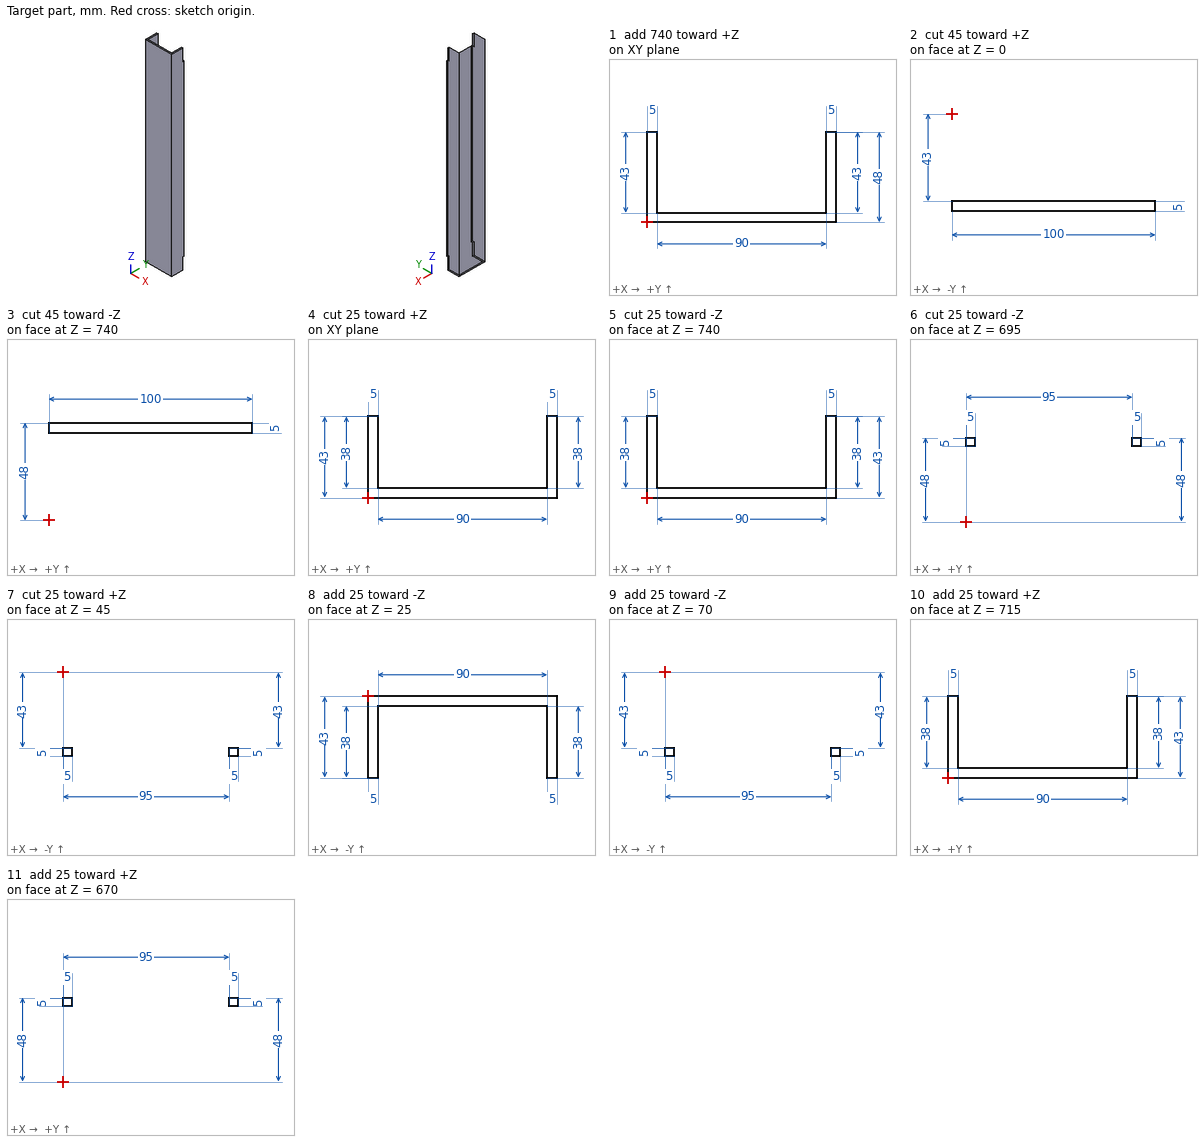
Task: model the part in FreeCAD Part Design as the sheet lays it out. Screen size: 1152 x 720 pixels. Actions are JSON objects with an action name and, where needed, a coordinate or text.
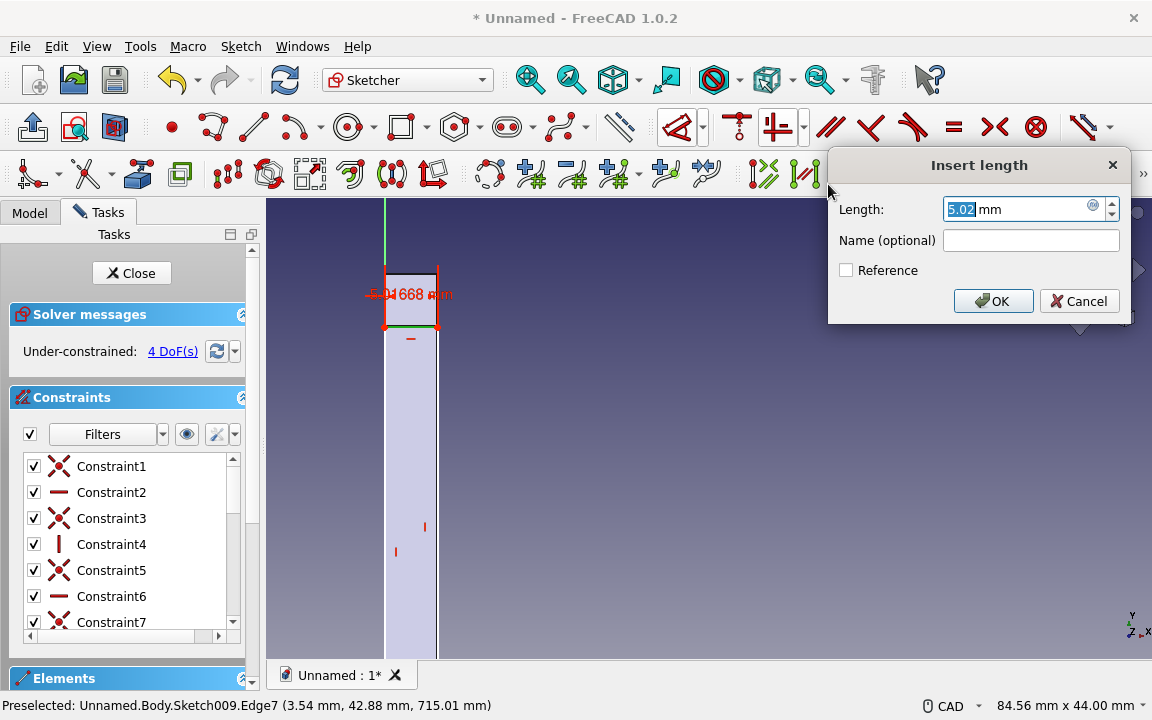
{"action": "type", "text": "5"}
{"action": "key", "text": "Return"}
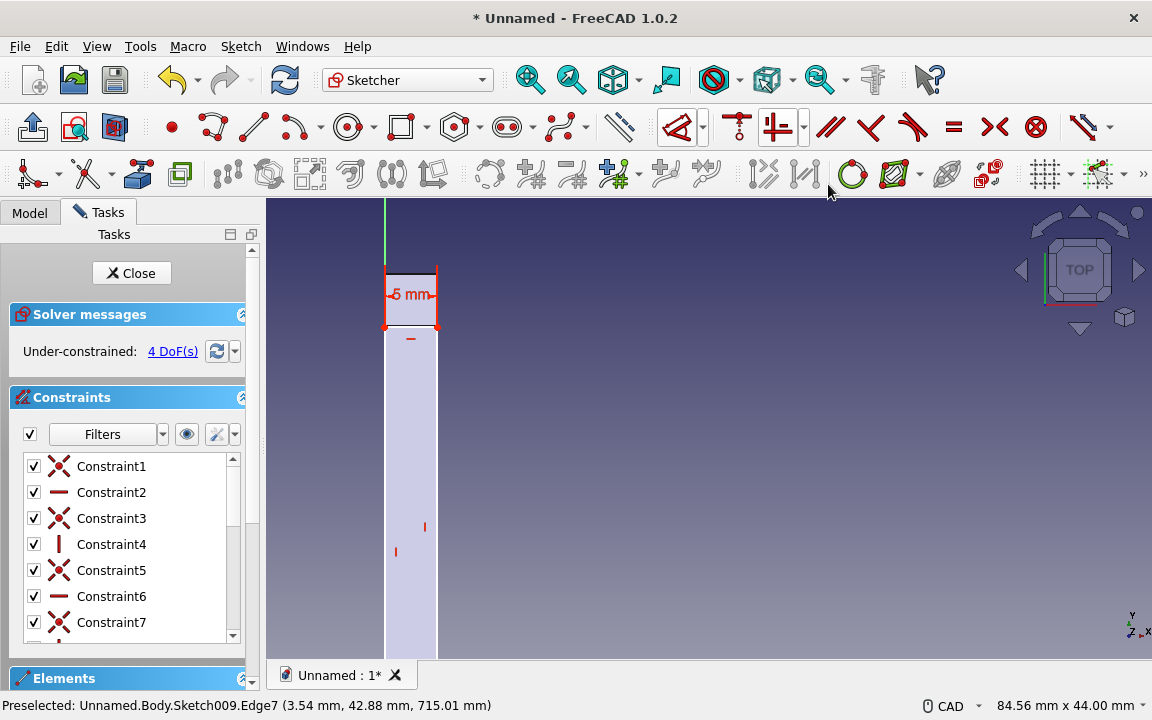
{"action": "scroll", "coordinate": [422, 328], "scroll_direction": "down", "scroll_amount": 4}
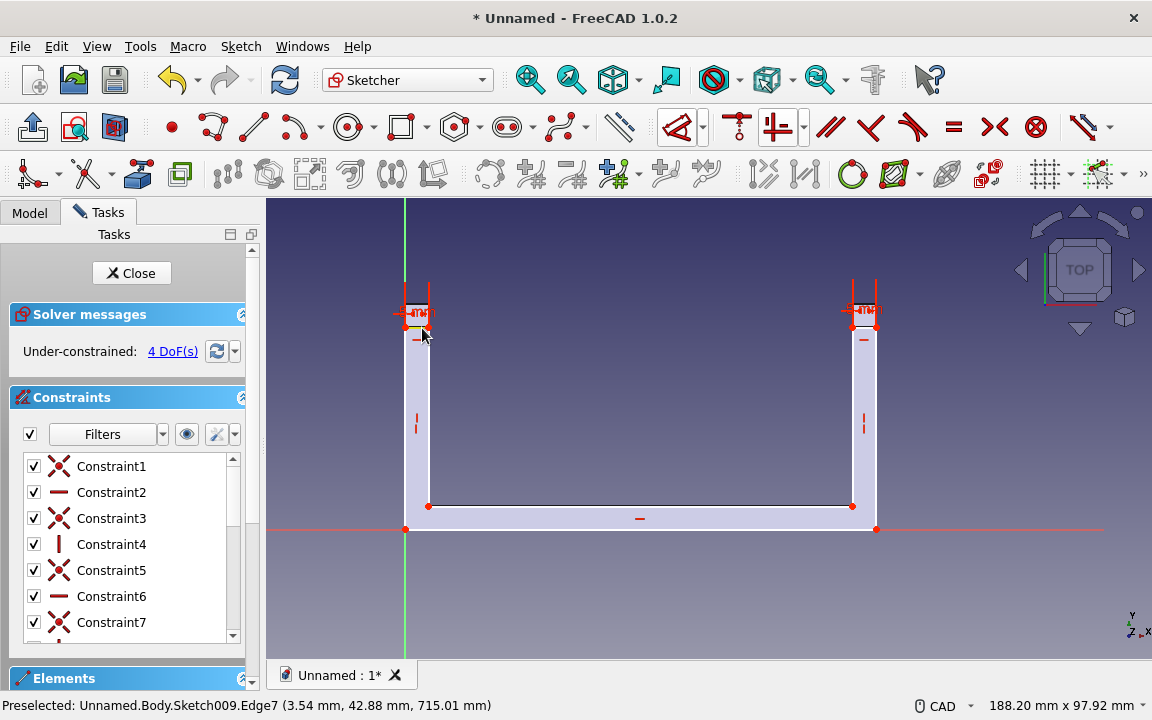
{"action": "left_click", "coordinate": [876, 469]}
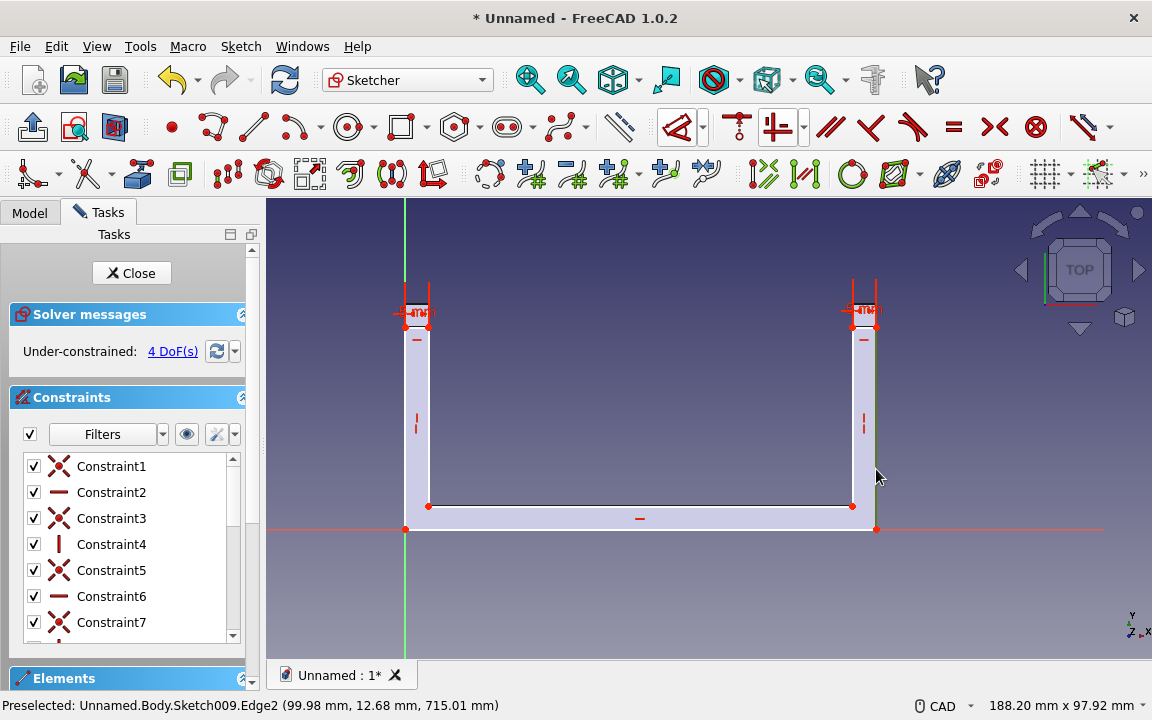
{"action": "left_click", "coordinate": [702, 128]}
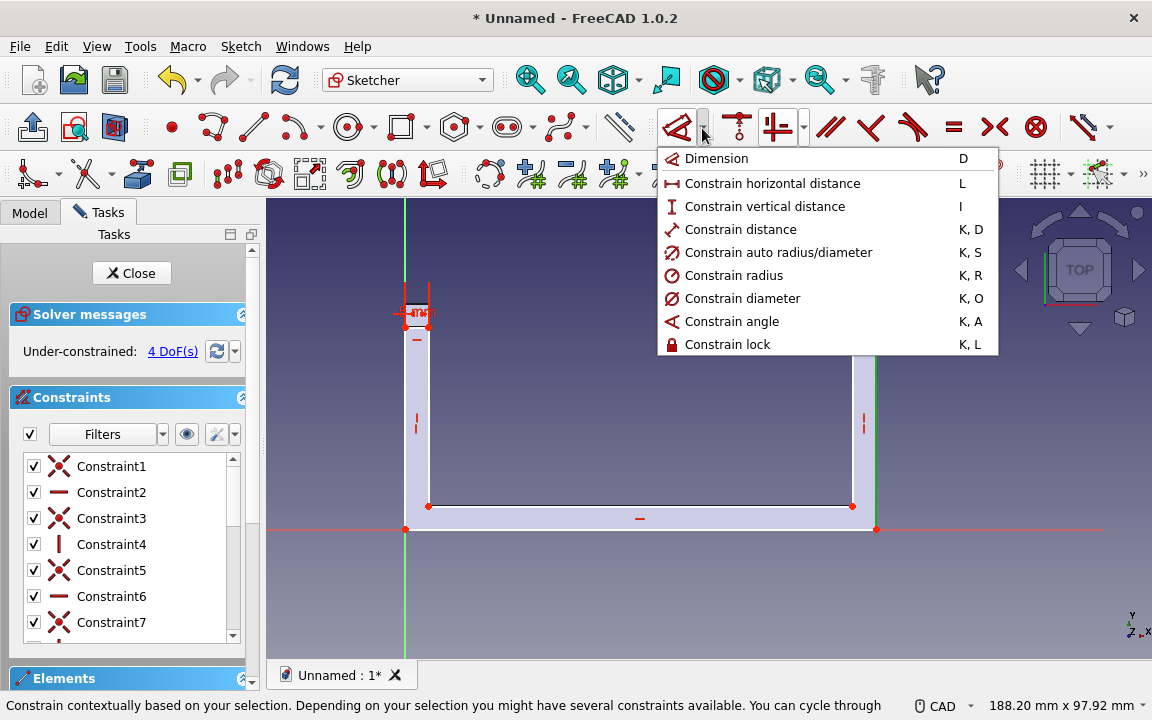
{"action": "left_click", "coordinate": [828, 206]}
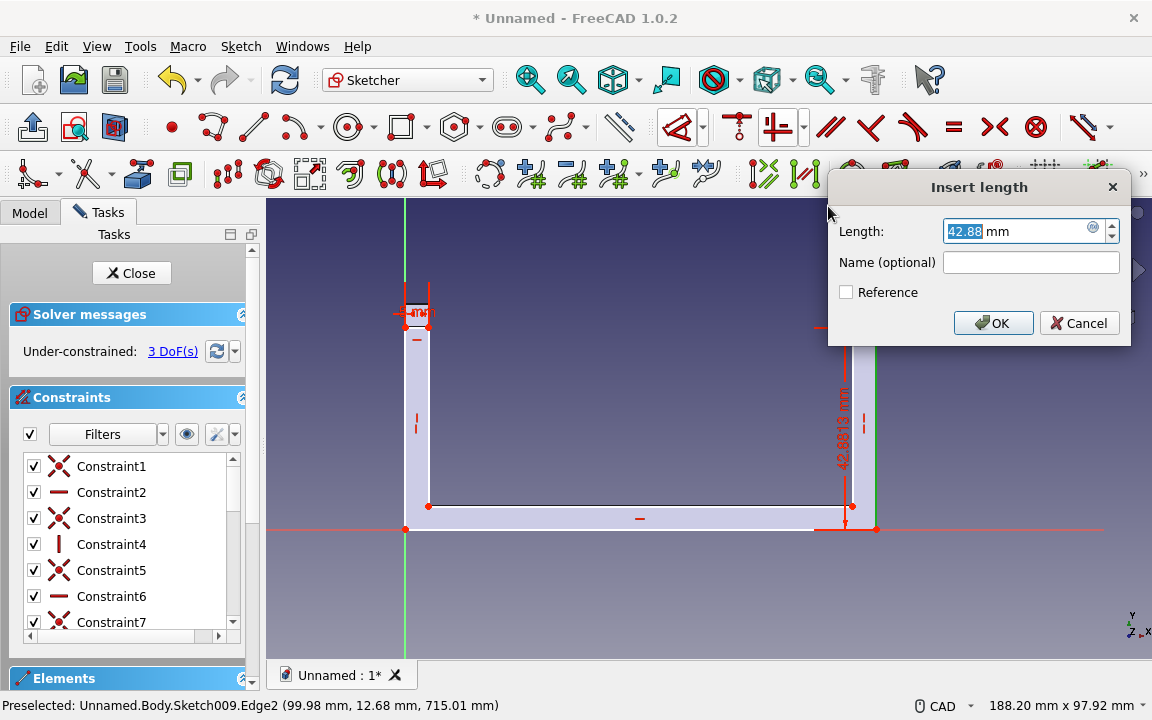
{"action": "type", "text": "43"}
{"action": "key", "text": "Return"}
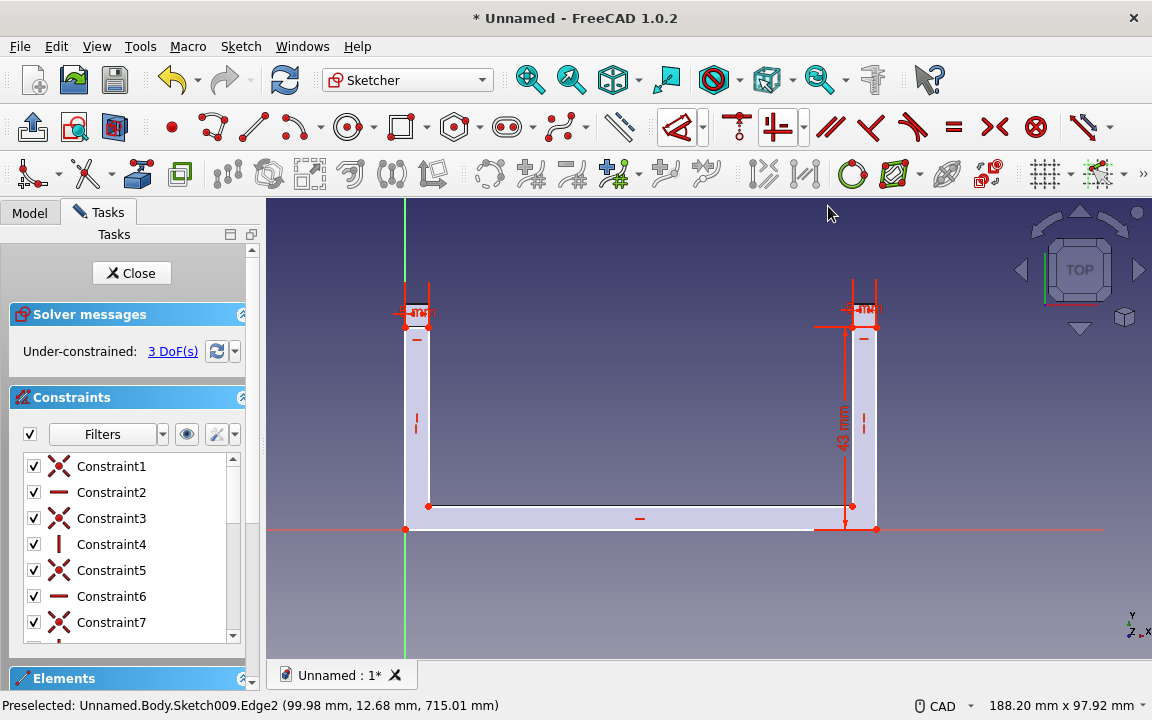
{"action": "left_click", "coordinate": [853, 381]}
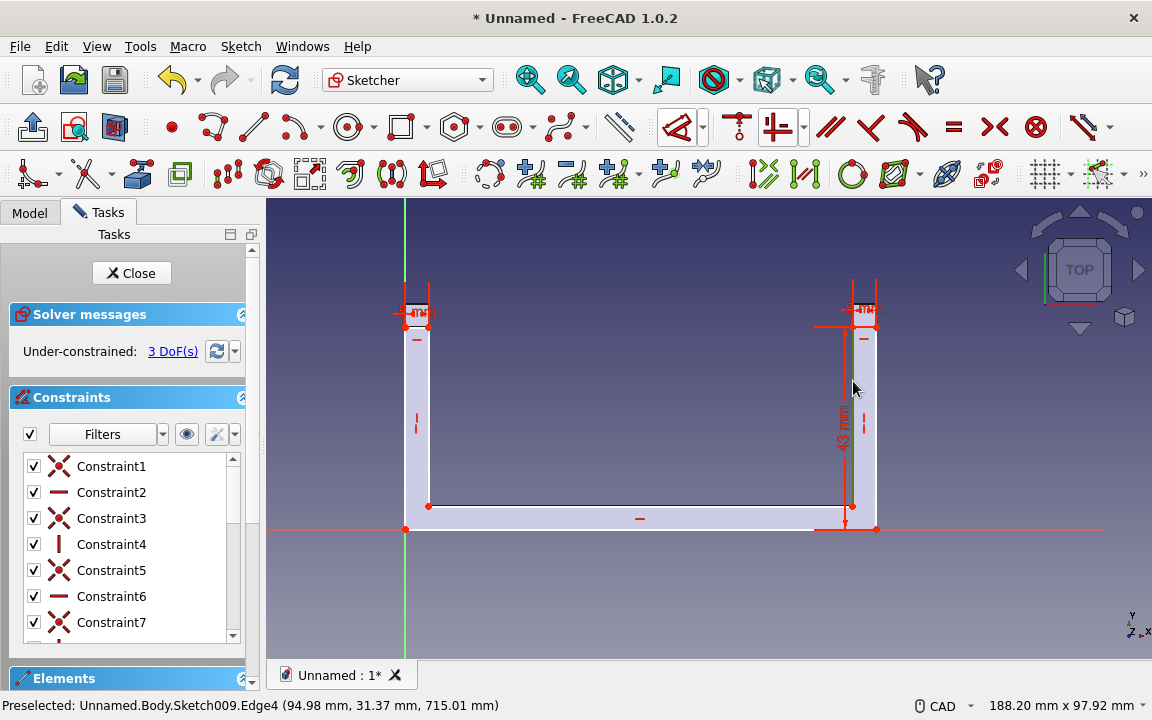
{"action": "key", "text": "i"}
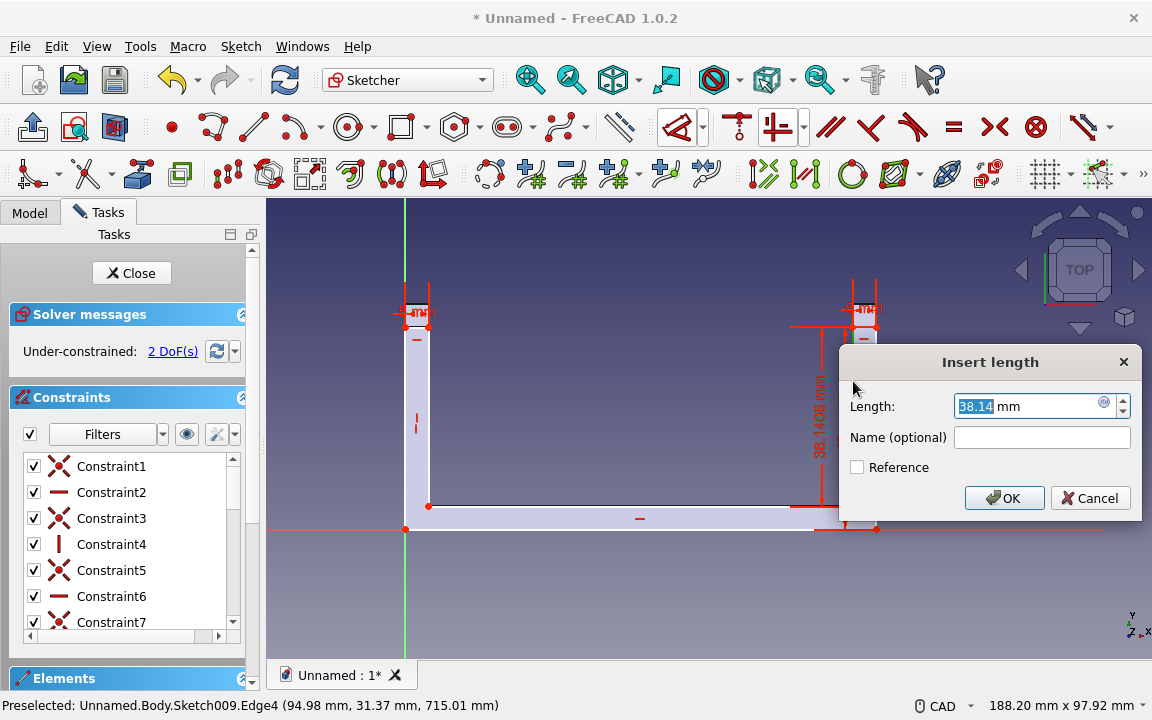
{"action": "type", "text": "38"}
{"action": "key", "text": "Return"}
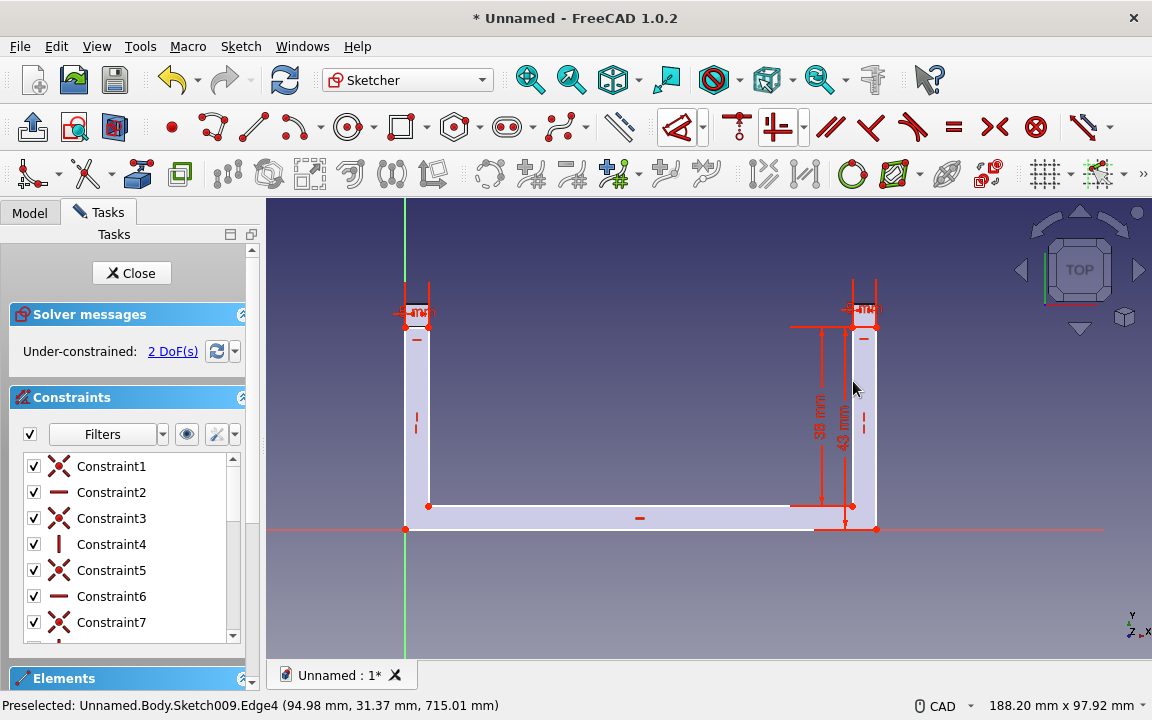
{"action": "left_click", "coordinate": [726, 506]}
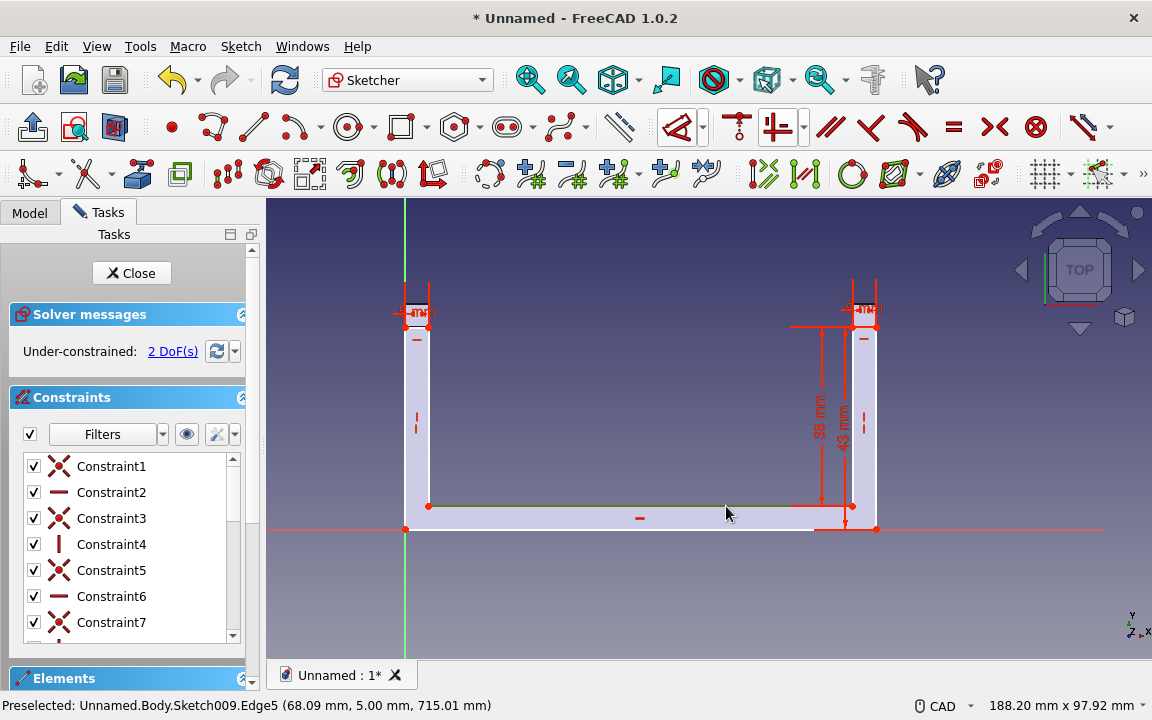
{"action": "key", "text": "l"}